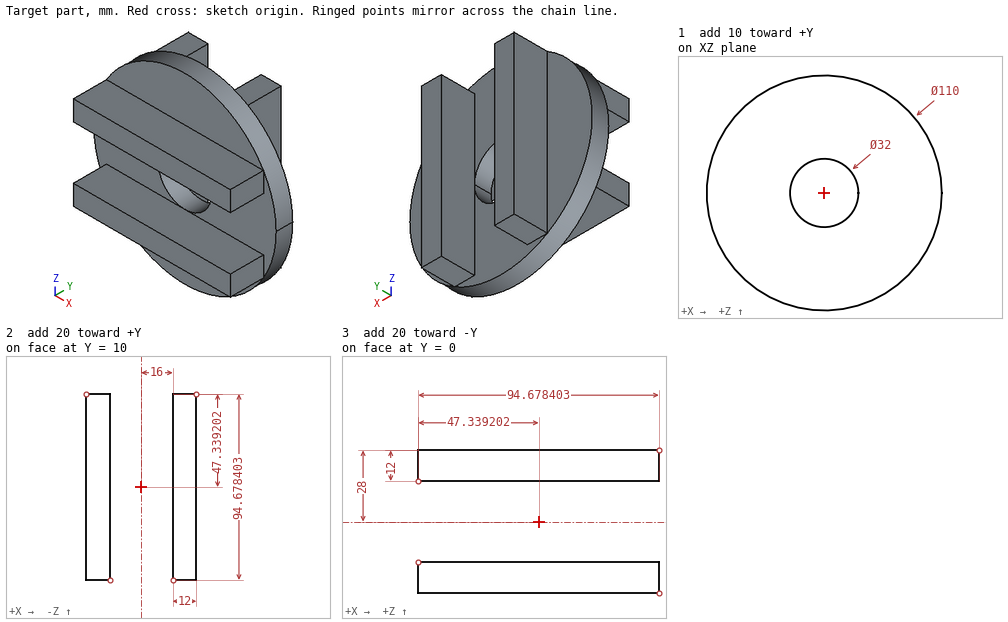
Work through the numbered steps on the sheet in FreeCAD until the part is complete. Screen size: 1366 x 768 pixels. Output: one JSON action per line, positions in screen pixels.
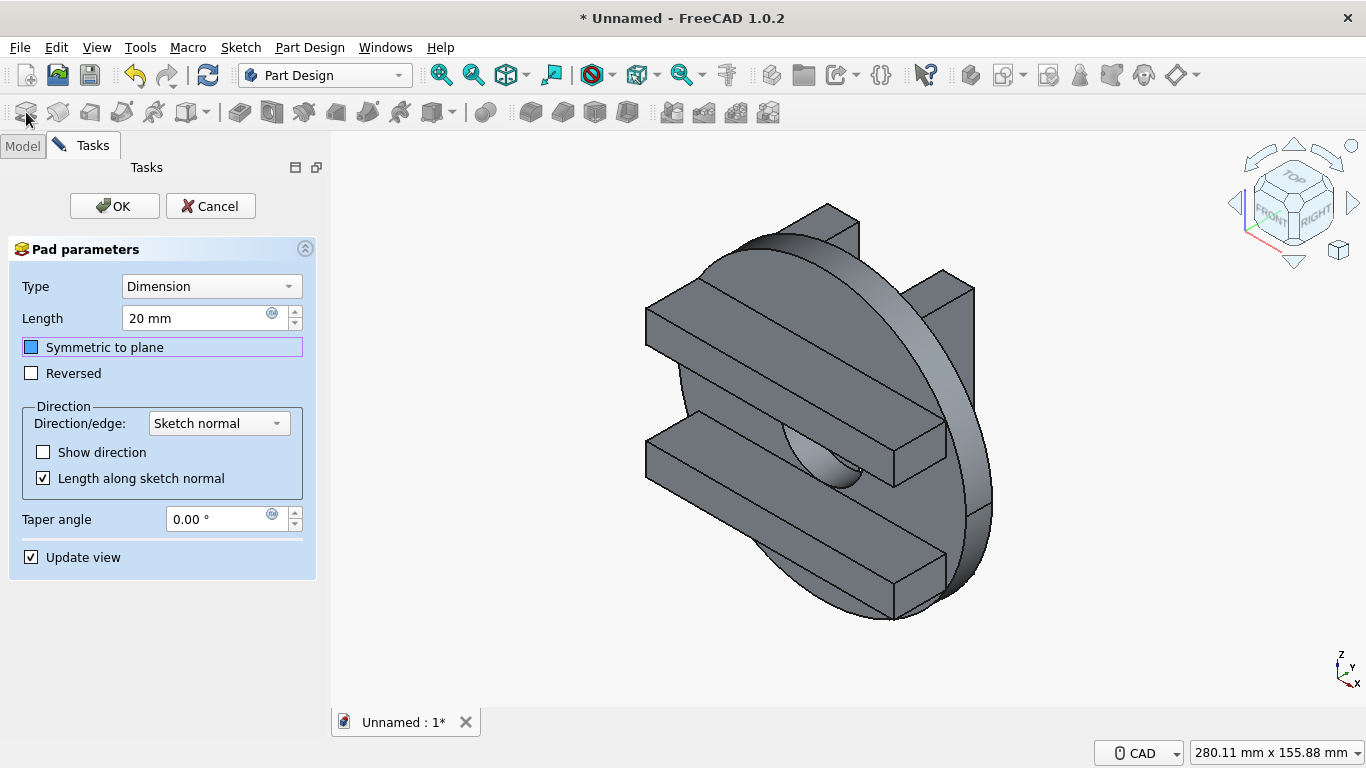
{"action": "left_click", "coordinate": [115, 206]}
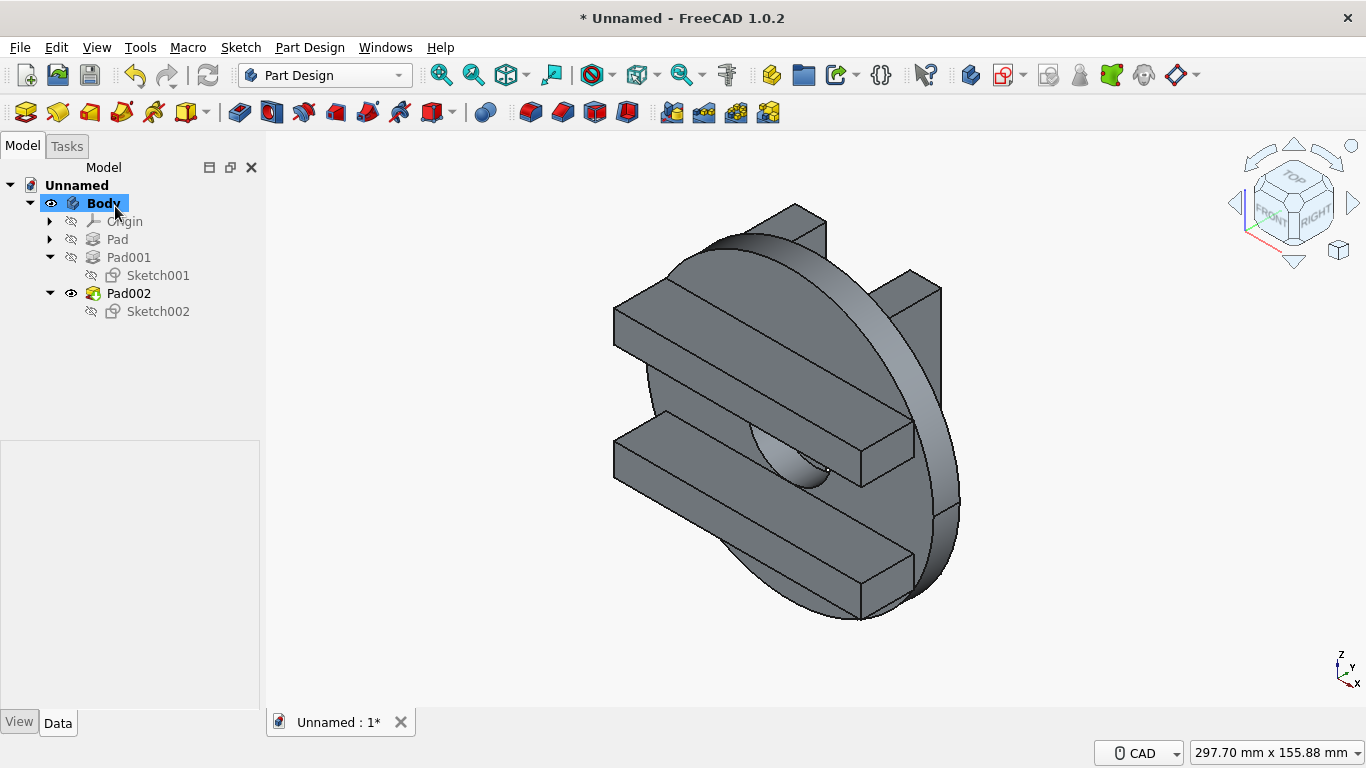
{"action": "key", "text": "v f"}